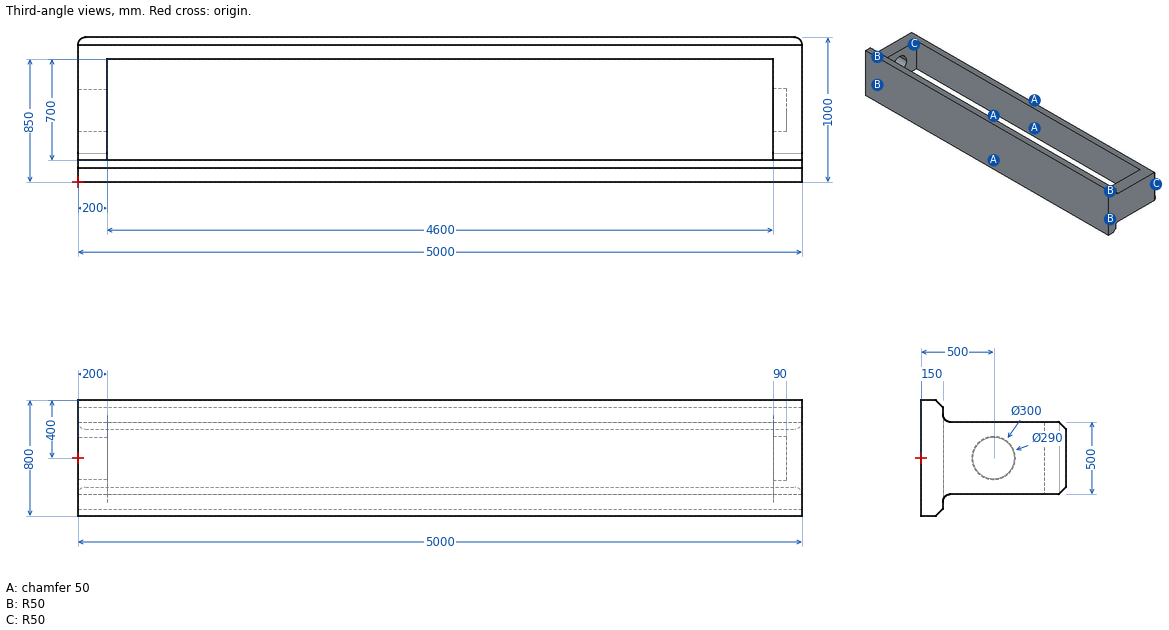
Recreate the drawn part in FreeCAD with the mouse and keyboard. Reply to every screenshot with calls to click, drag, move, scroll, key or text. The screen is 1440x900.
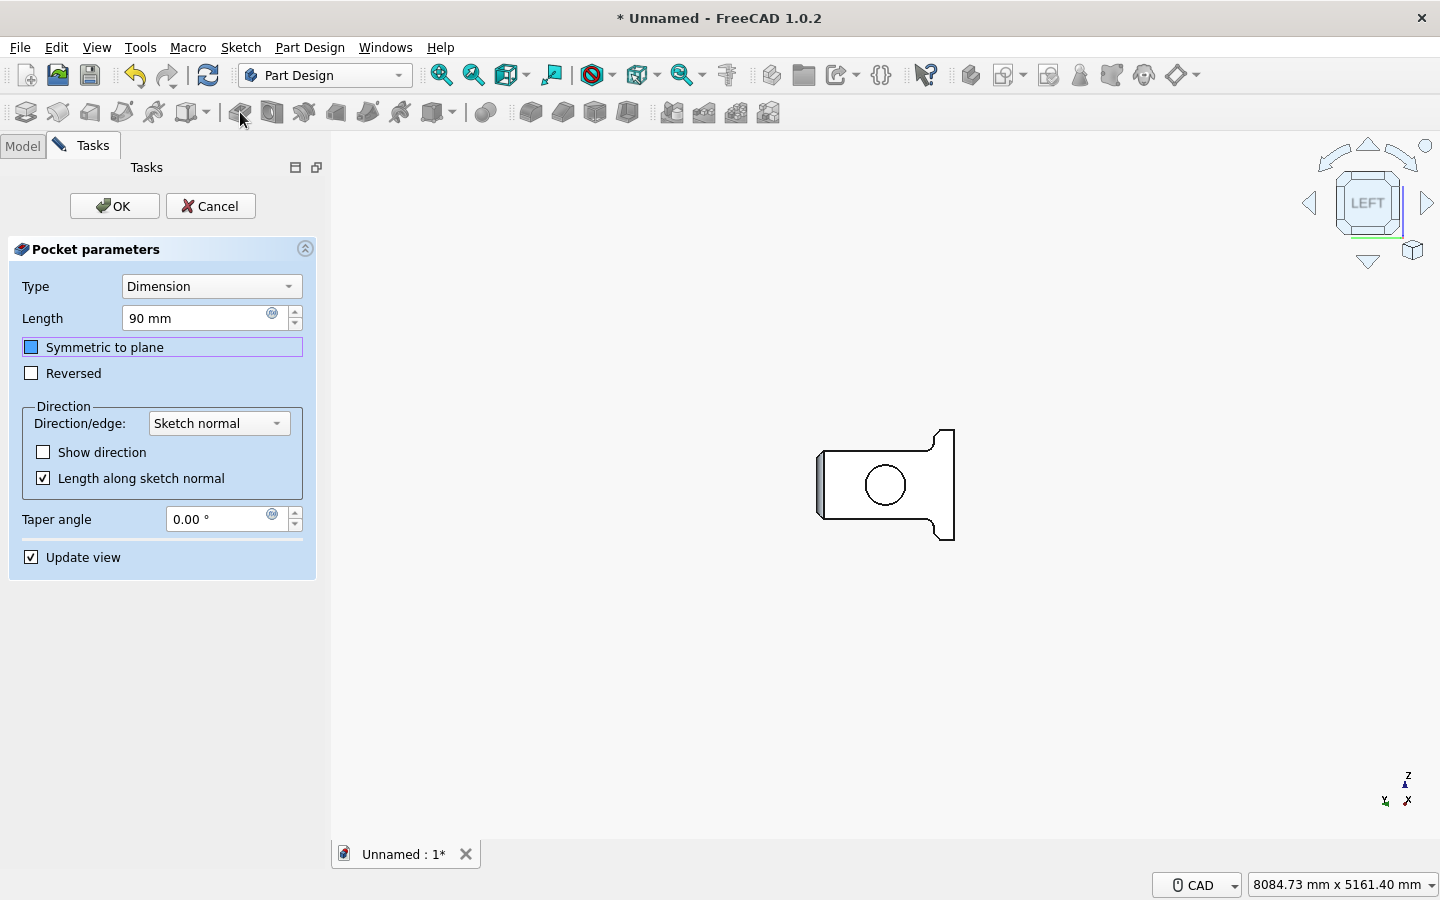
click(115, 206)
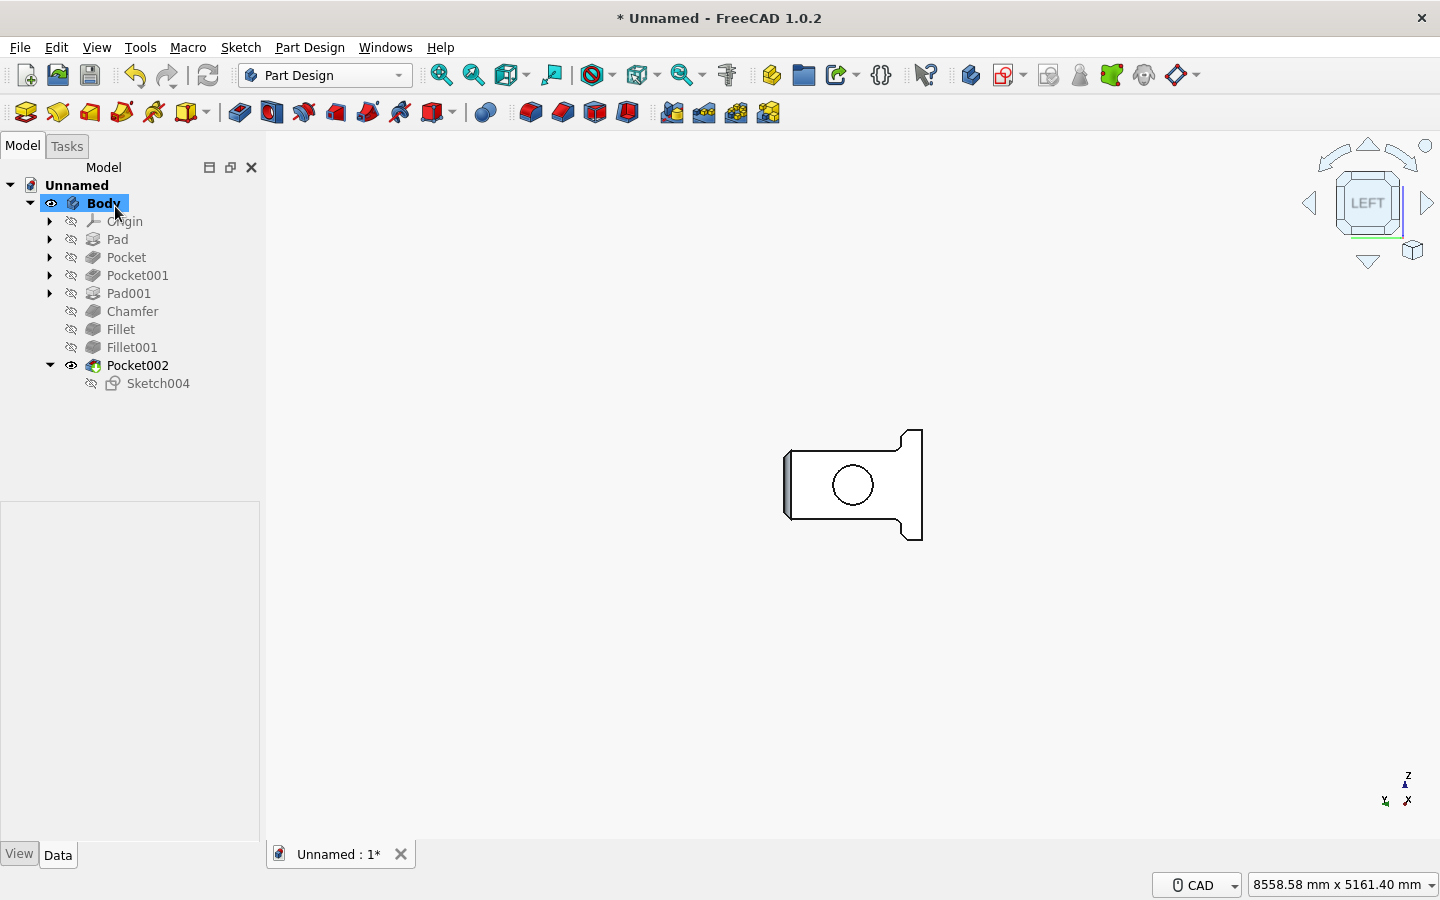
key(0)